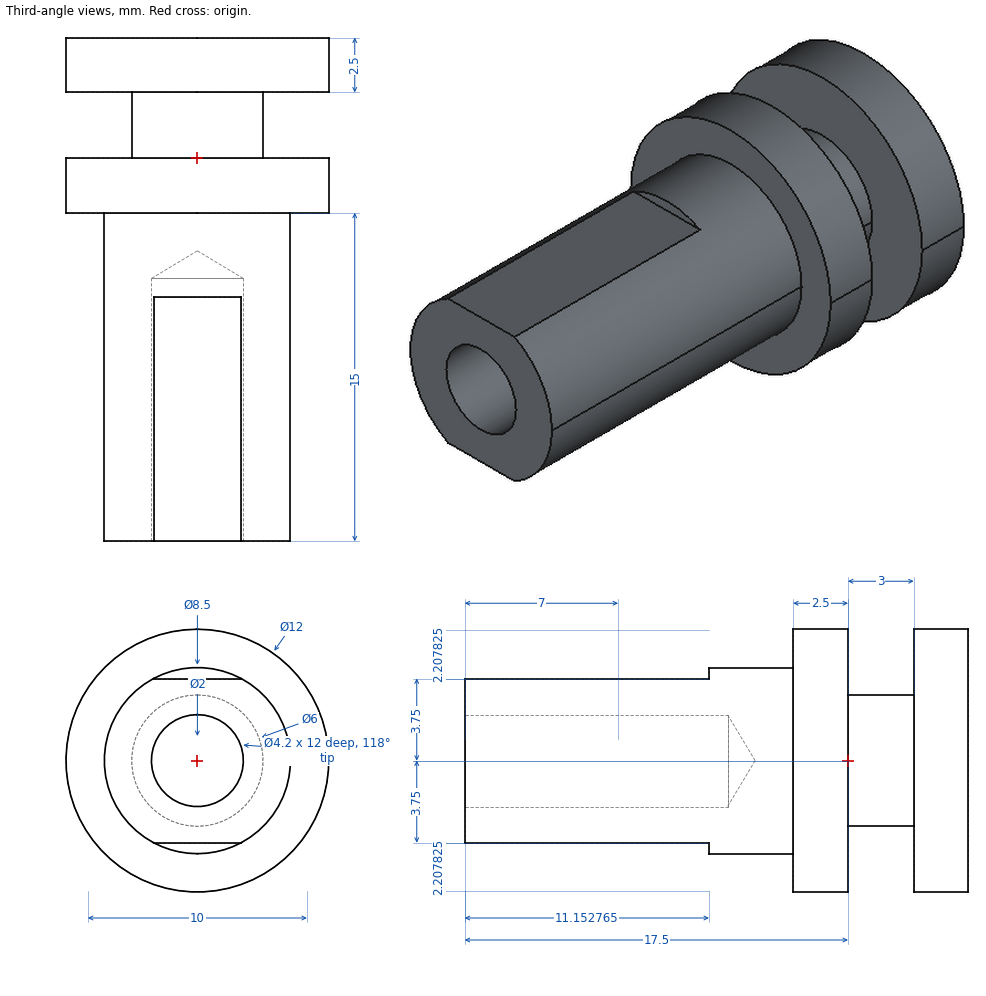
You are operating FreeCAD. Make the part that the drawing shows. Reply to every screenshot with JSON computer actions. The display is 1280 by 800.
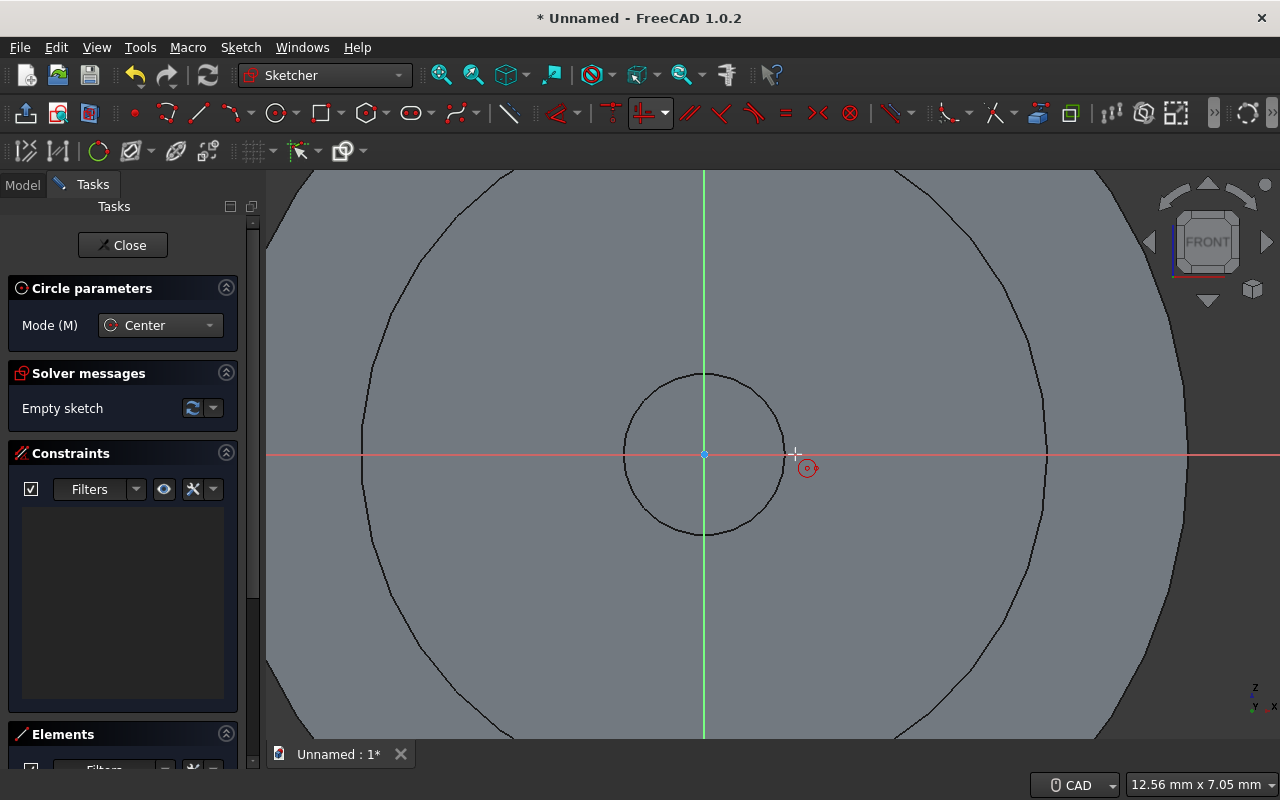
{"action": "left_click", "coordinate": [704, 454]}
{"action": "mouse_move", "coordinate": [824, 335]}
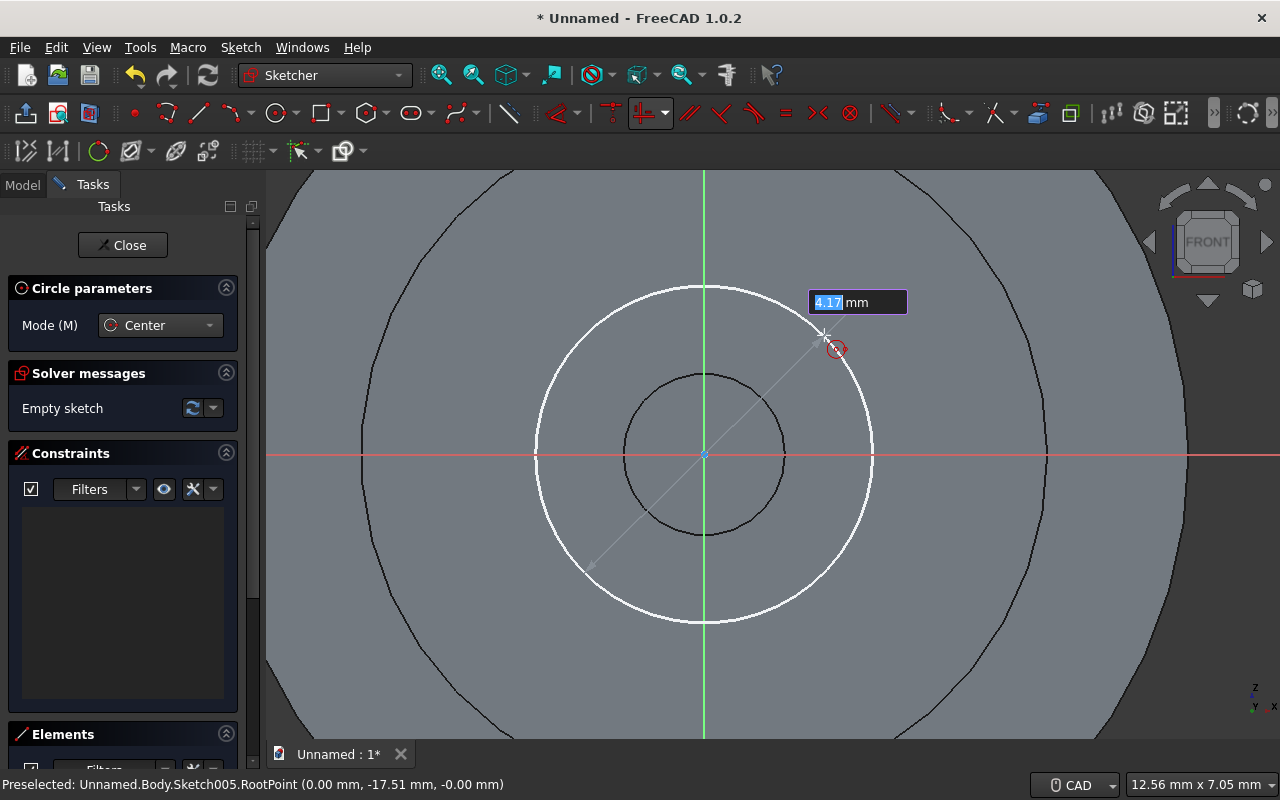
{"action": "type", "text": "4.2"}
{"action": "key", "text": "Return"}
{"action": "key", "text": "Escape"}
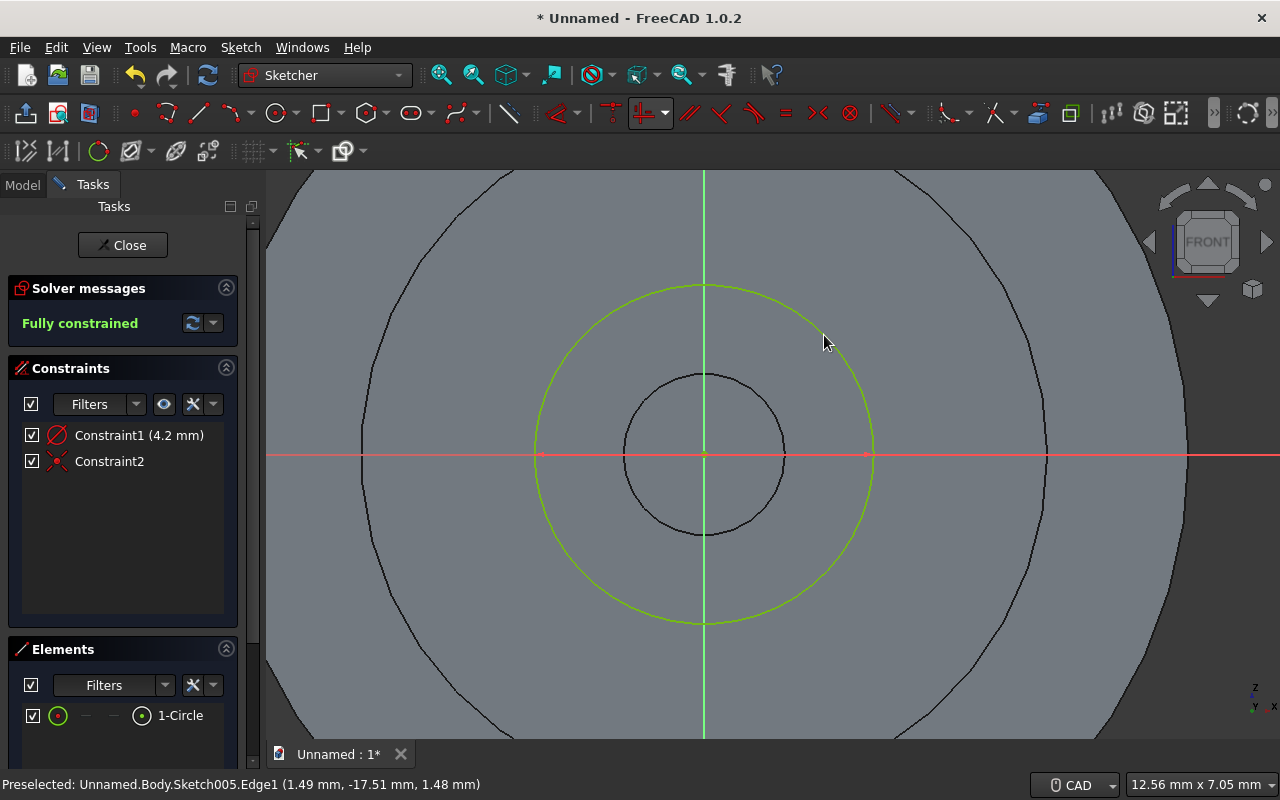
{"action": "left_click", "coordinate": [123, 245]}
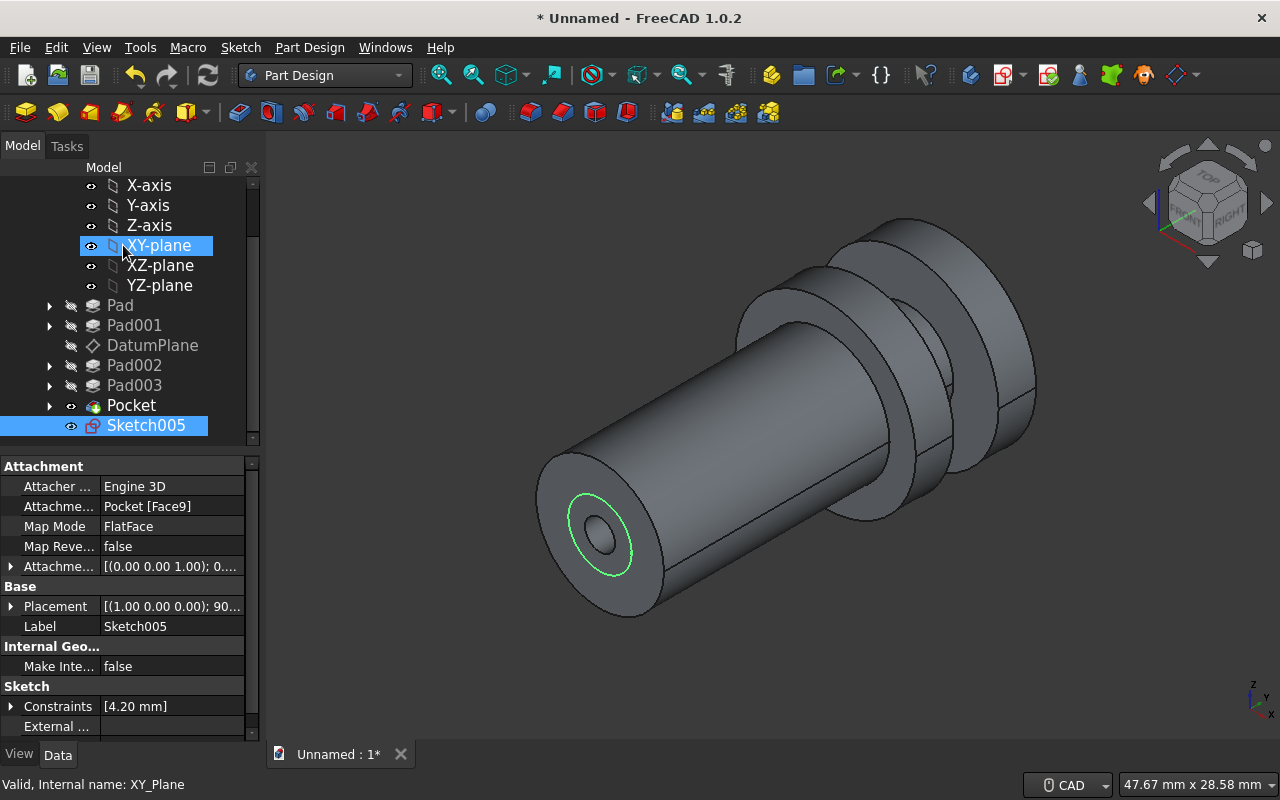
{"action": "left_click", "coordinate": [272, 112]}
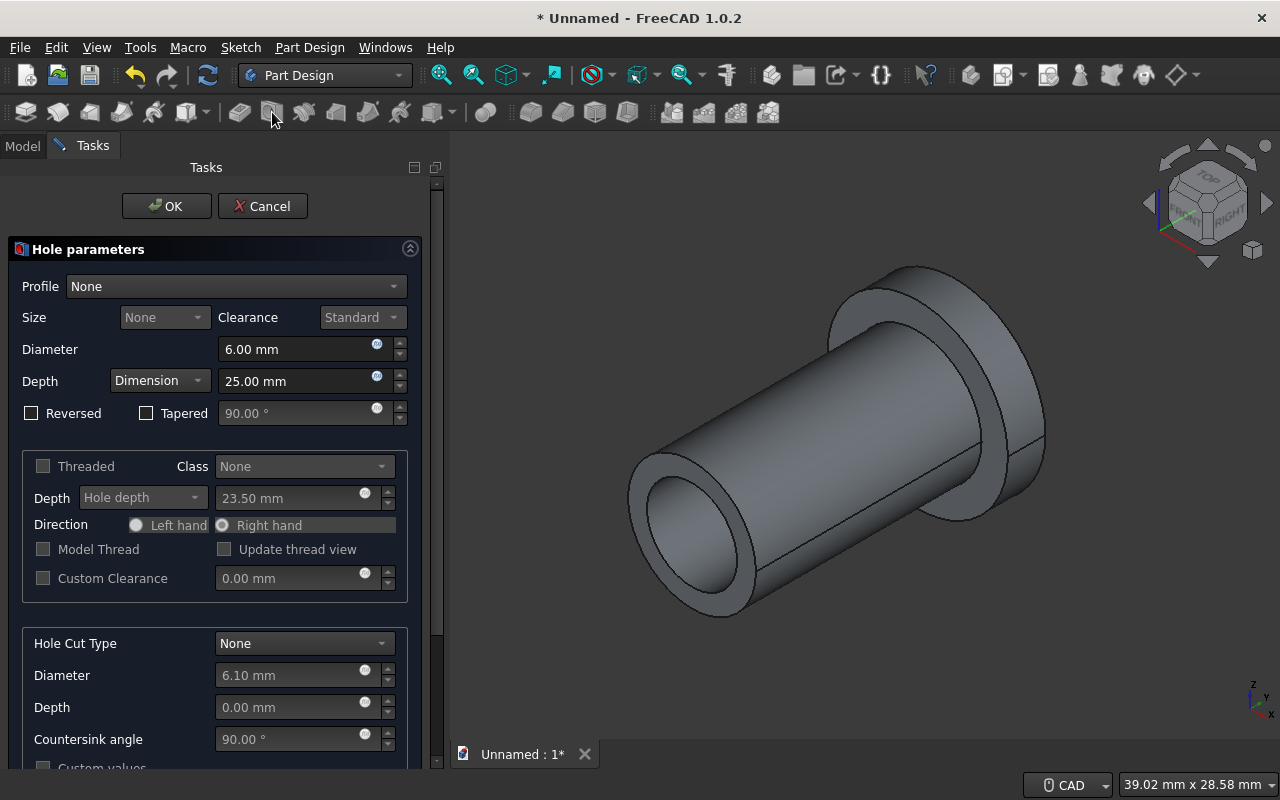
{"action": "triple_click", "coordinate": [305, 349]}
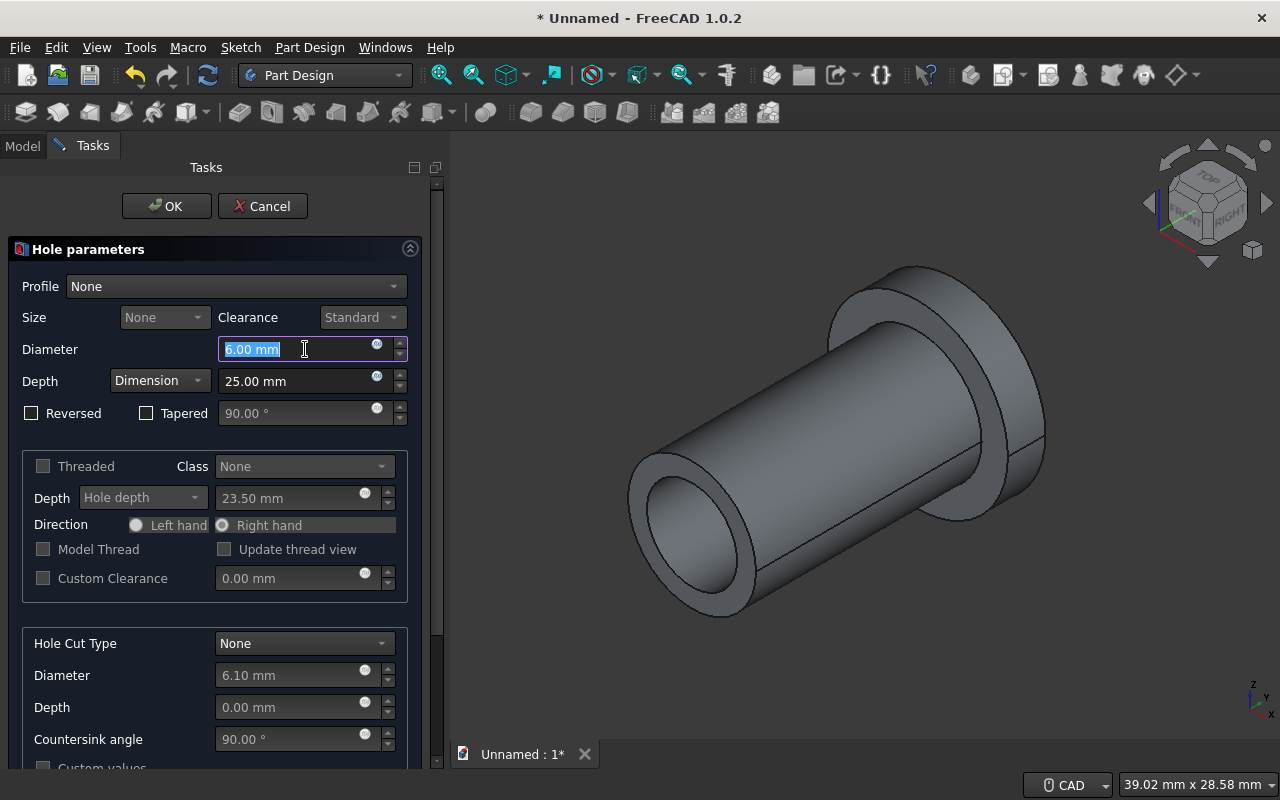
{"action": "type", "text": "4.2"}
{"action": "key", "text": "Tab"}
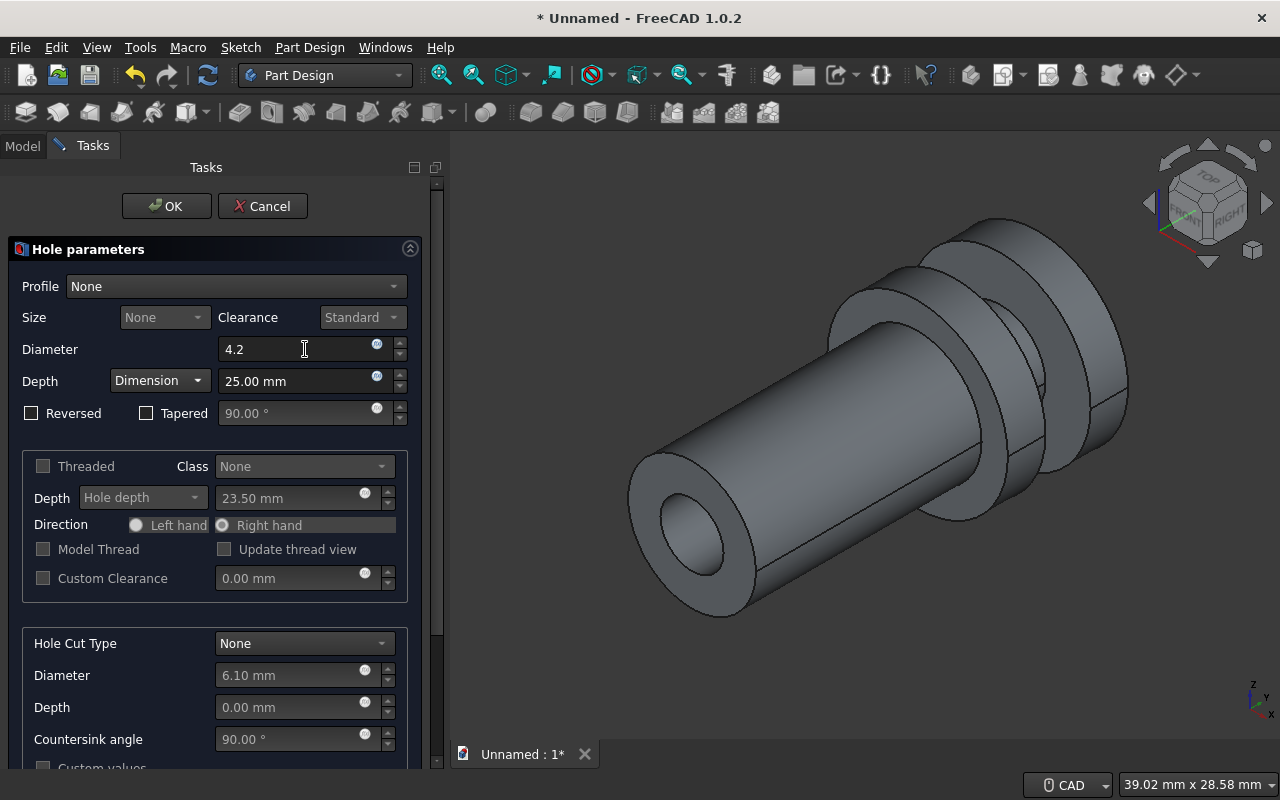
{"action": "triple_click", "coordinate": [305, 381]}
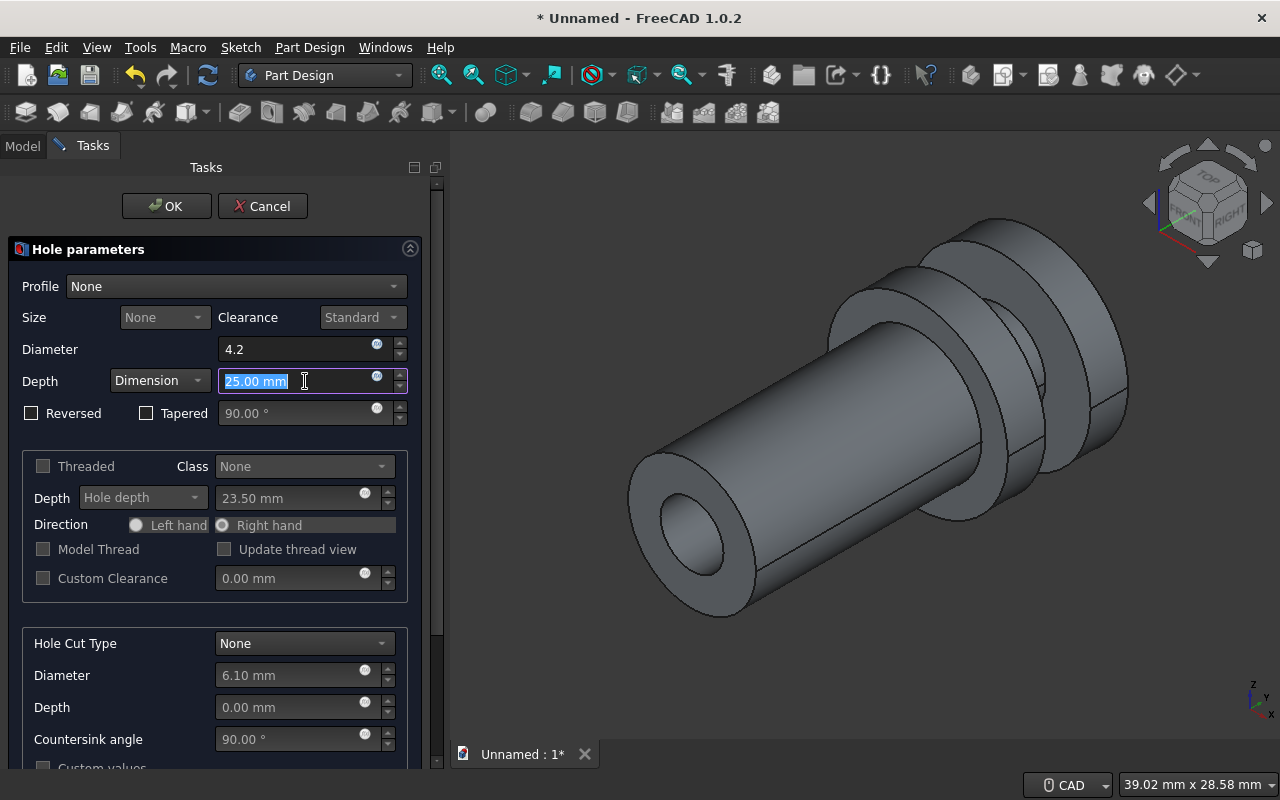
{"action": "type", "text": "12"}
{"action": "key", "text": "Tab"}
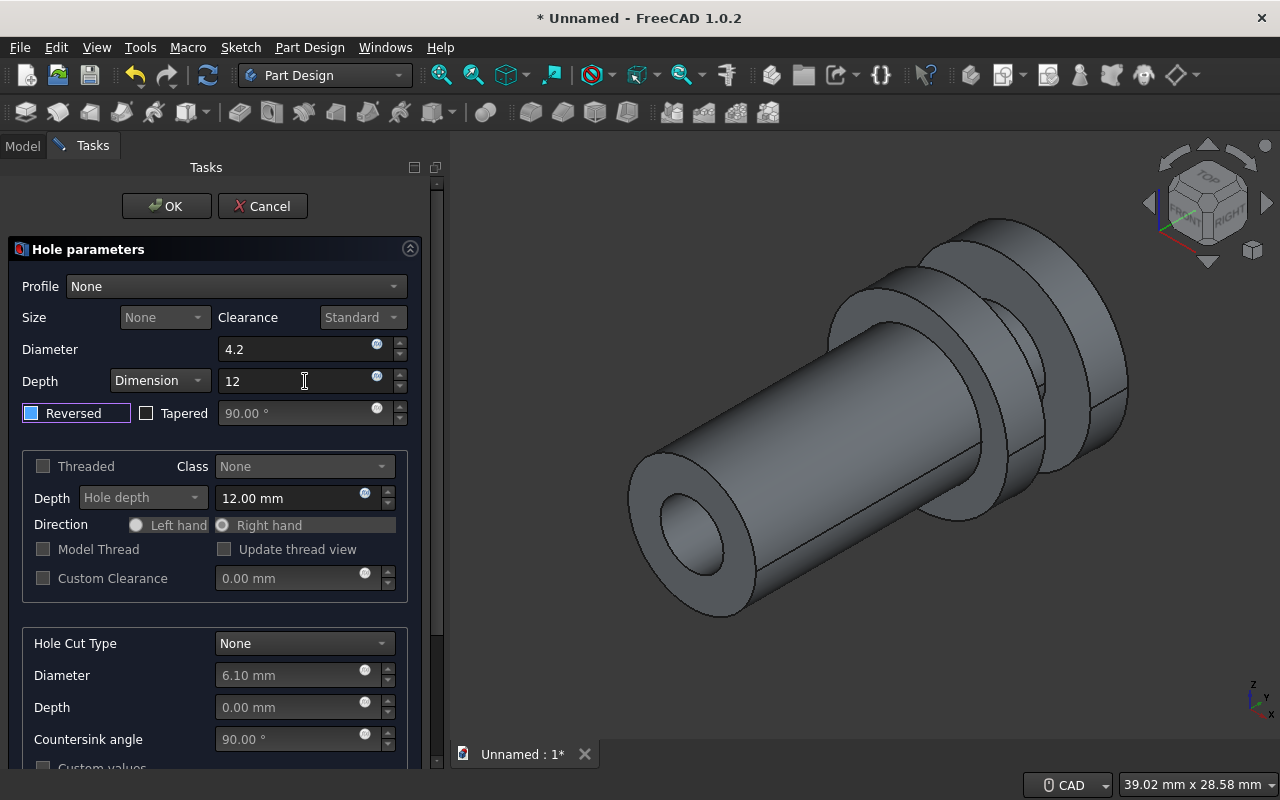
{"action": "left_click", "coordinate": [167, 206]}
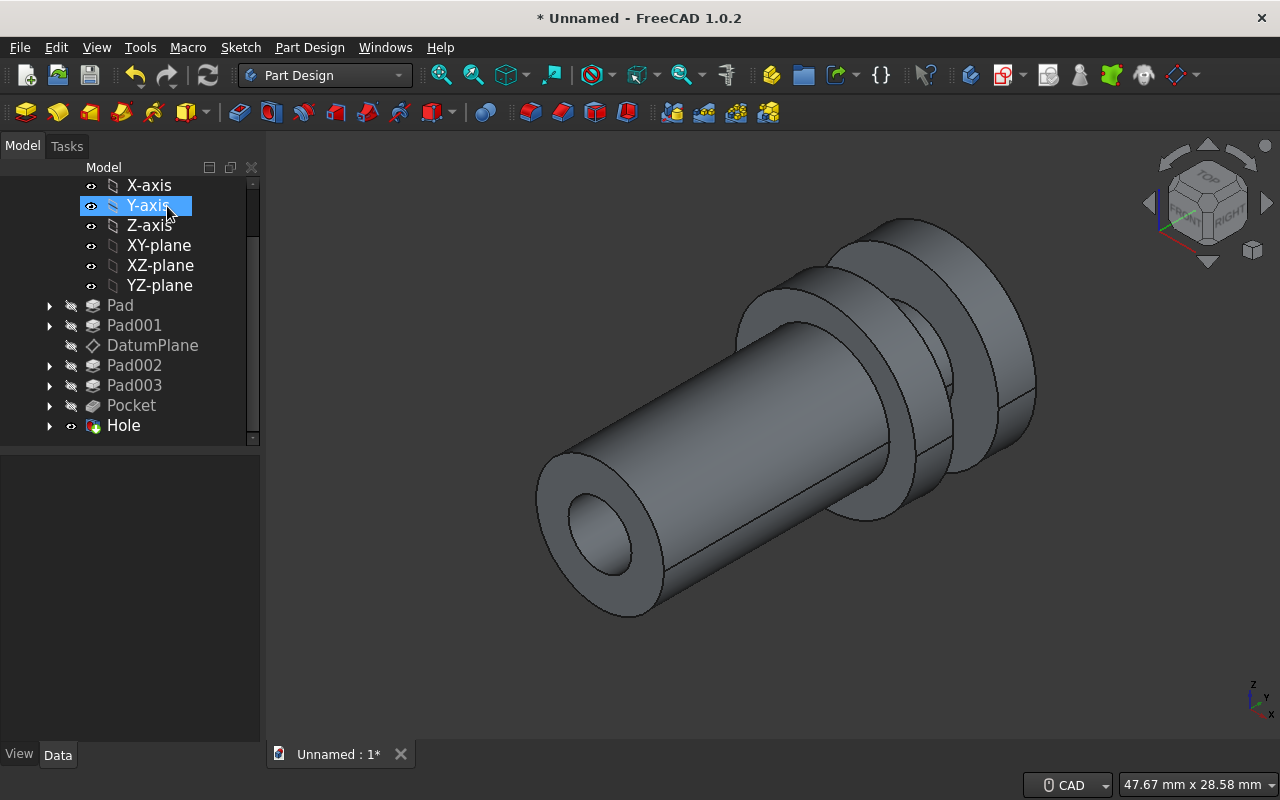
{"action": "left_click", "coordinate": [1004, 76]}